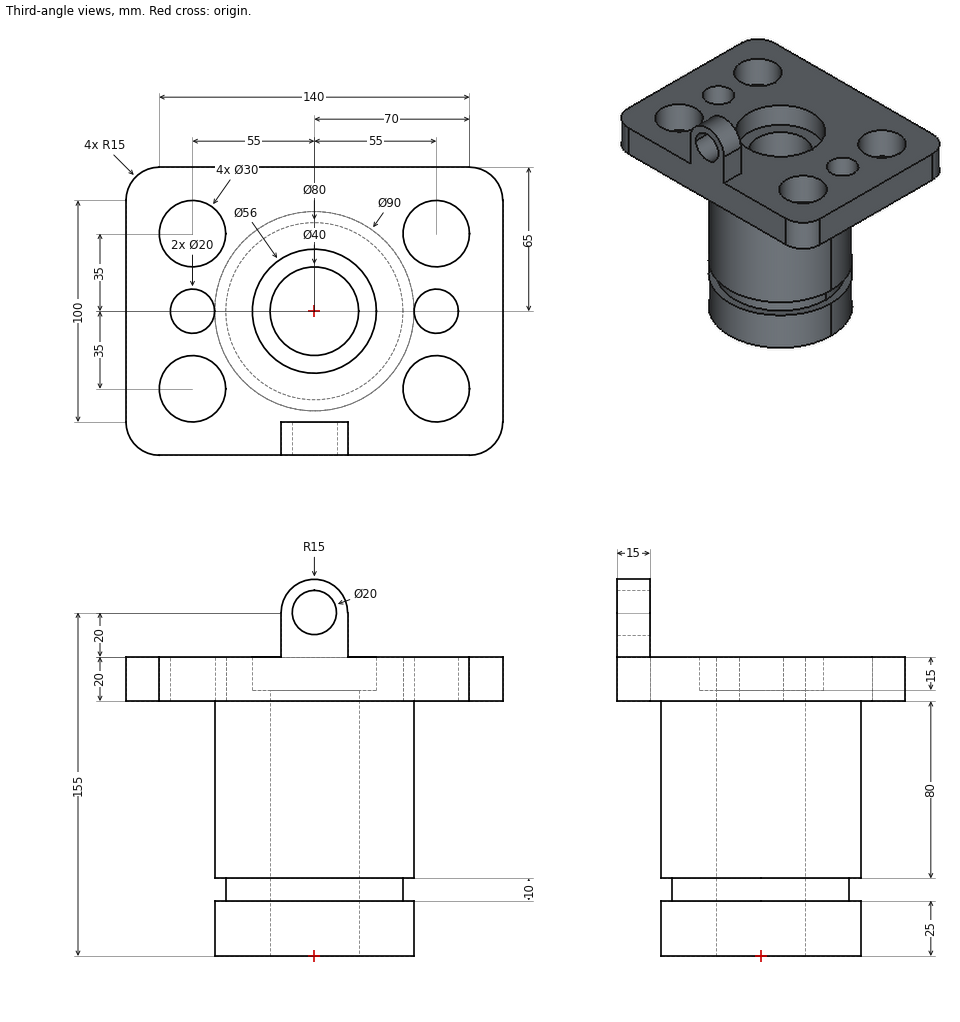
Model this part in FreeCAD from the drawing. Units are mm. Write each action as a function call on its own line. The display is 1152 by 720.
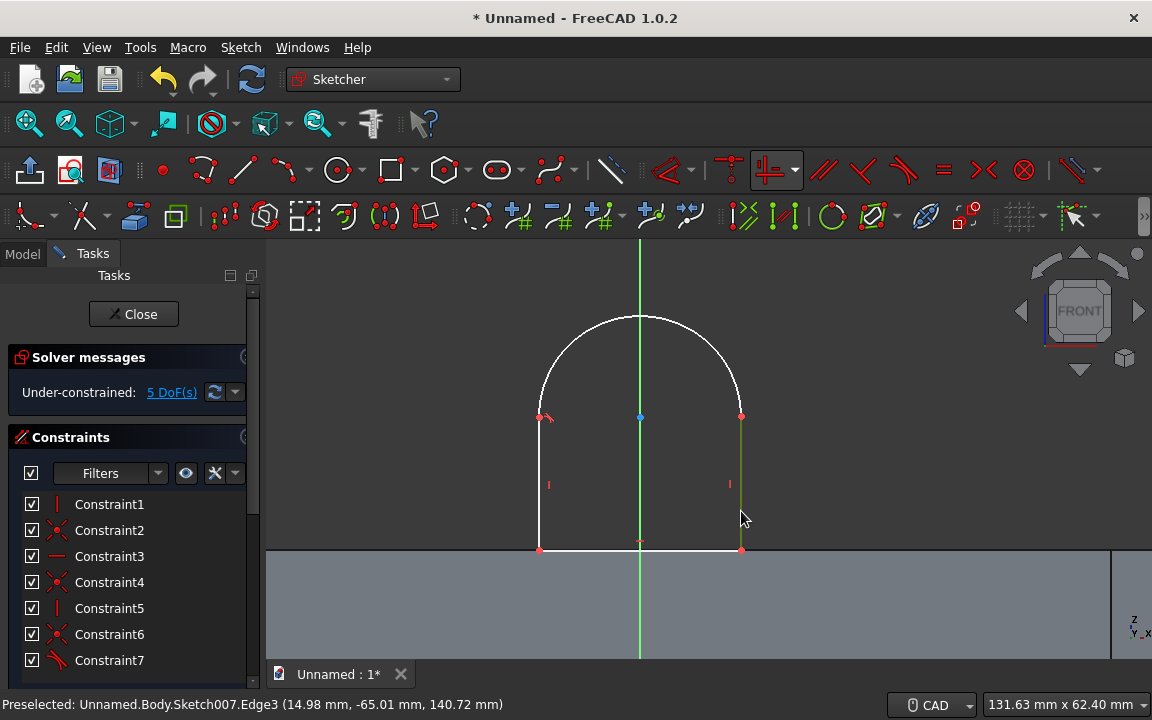
click(699, 335)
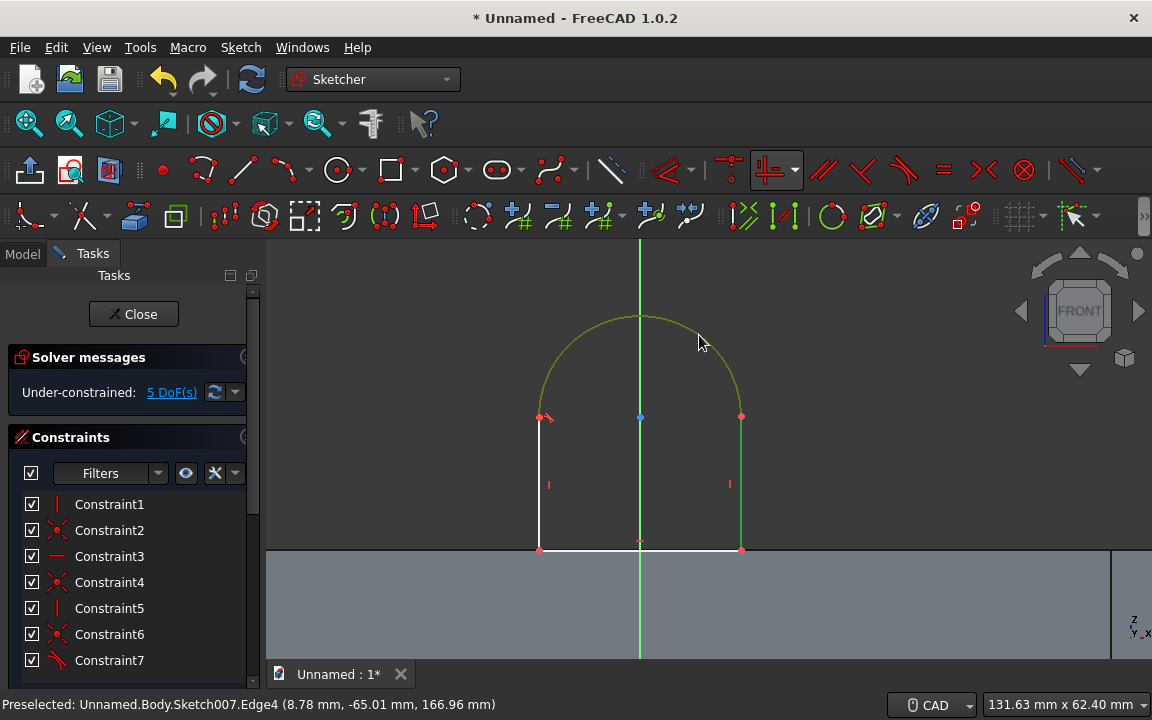
click(904, 170)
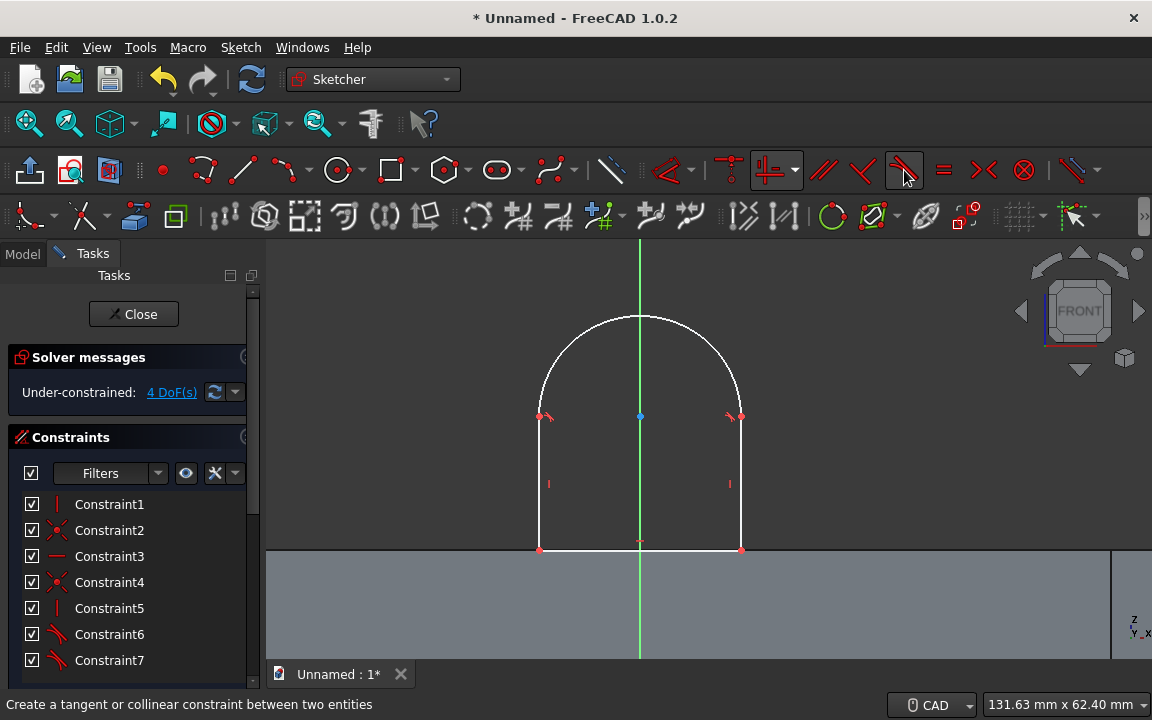
click(640, 417)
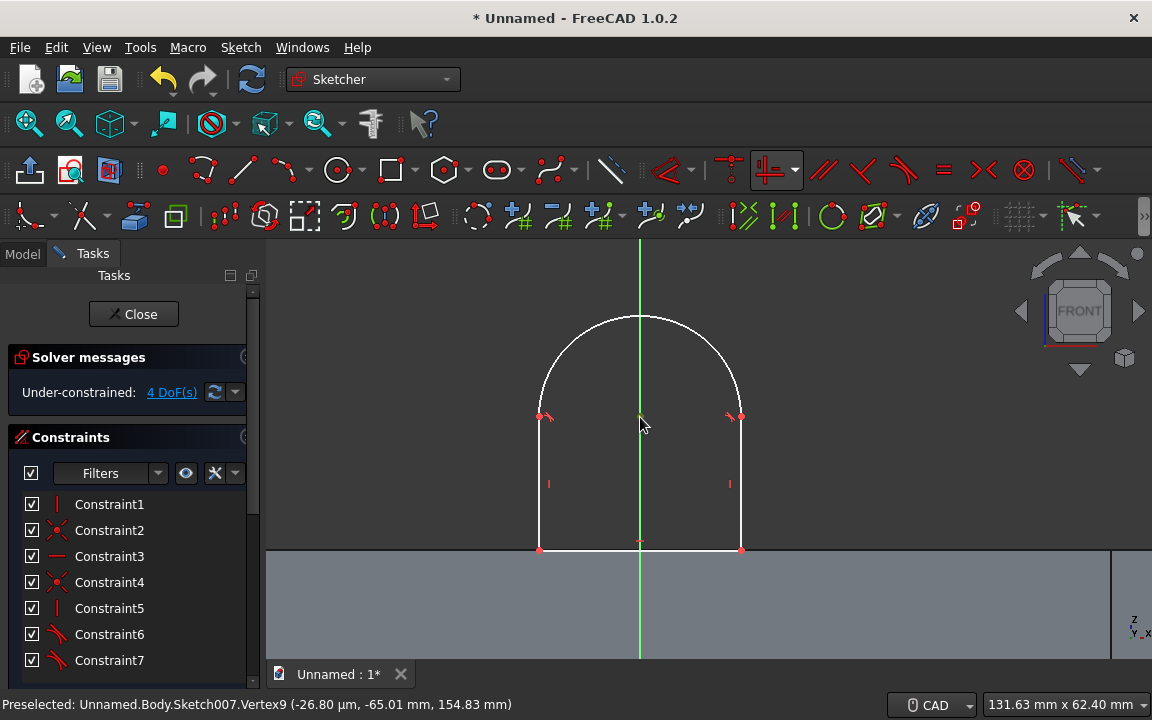
click(640, 605)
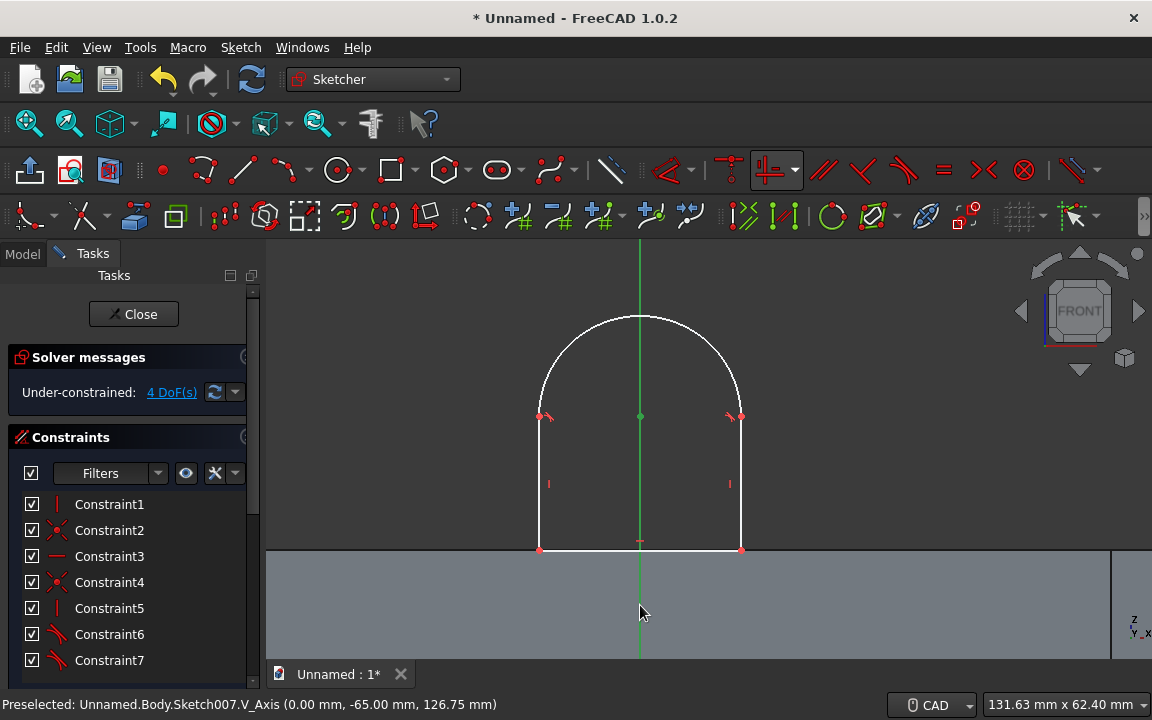
click(730, 170)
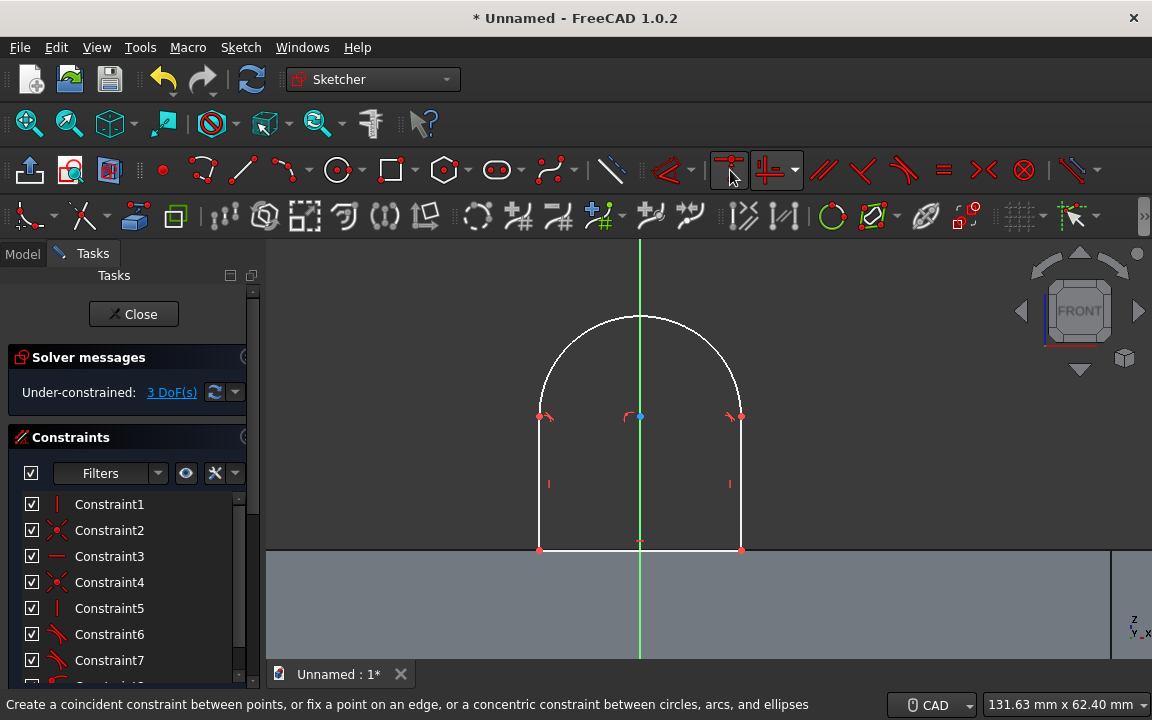
click(666, 170)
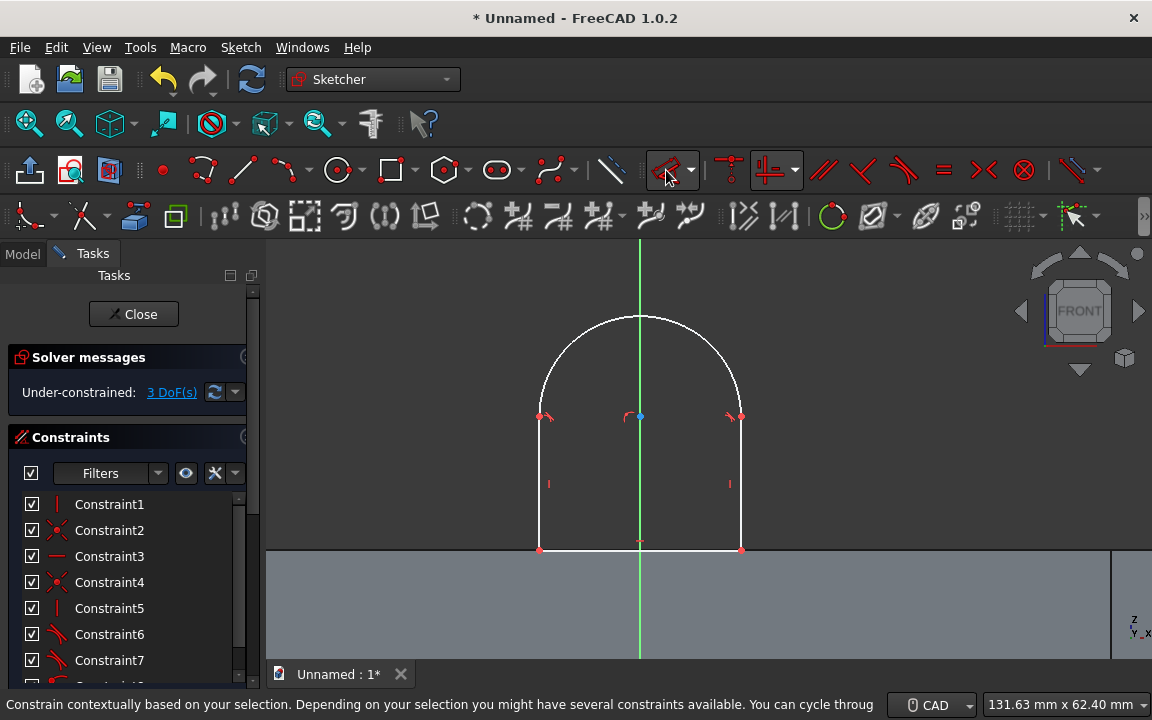
click(699, 335)
click(718, 309)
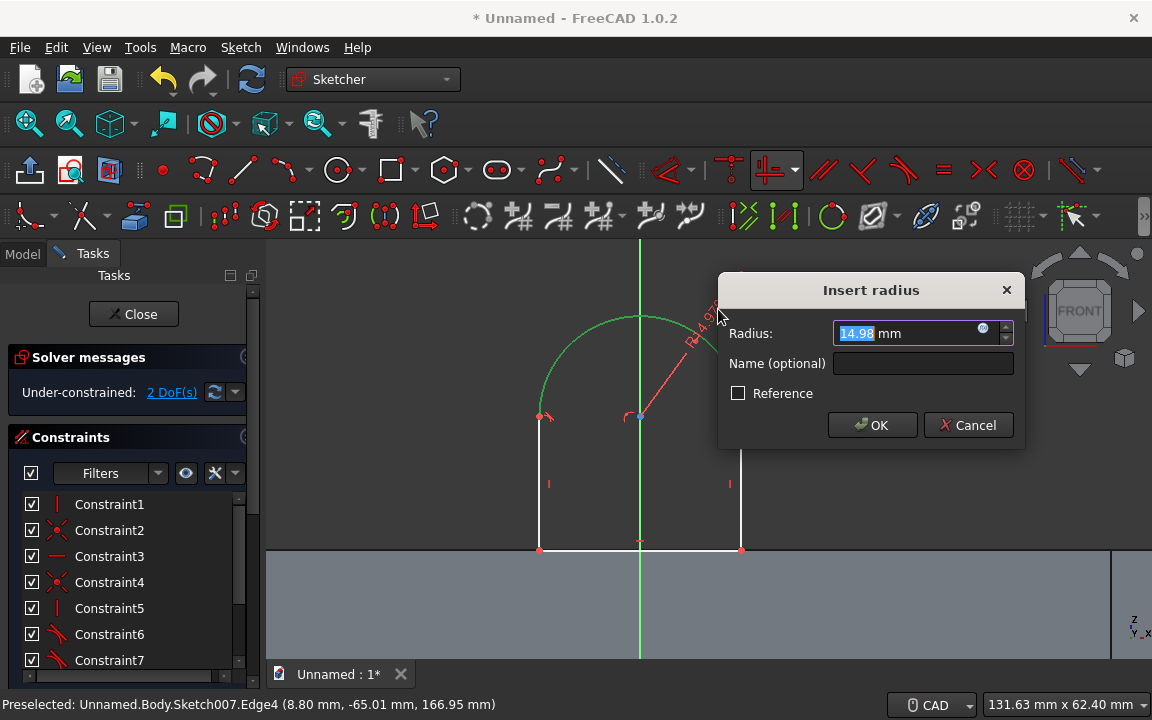
text(15)
key(Return)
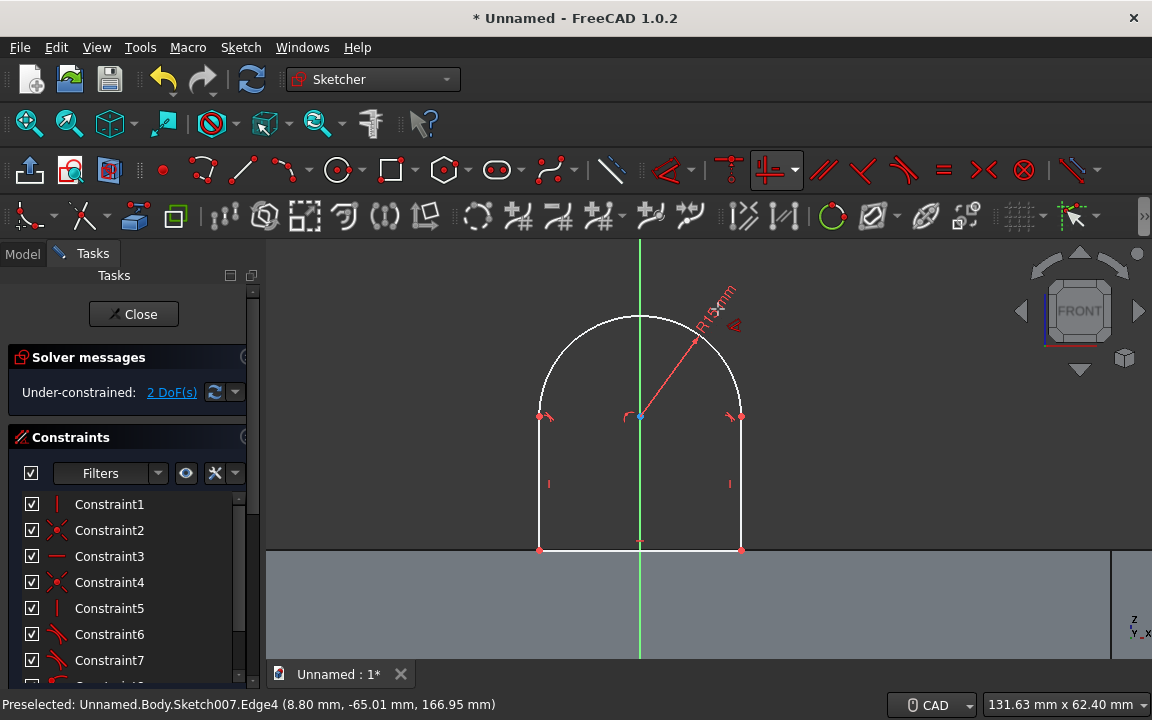
click(539, 457)
click(505, 484)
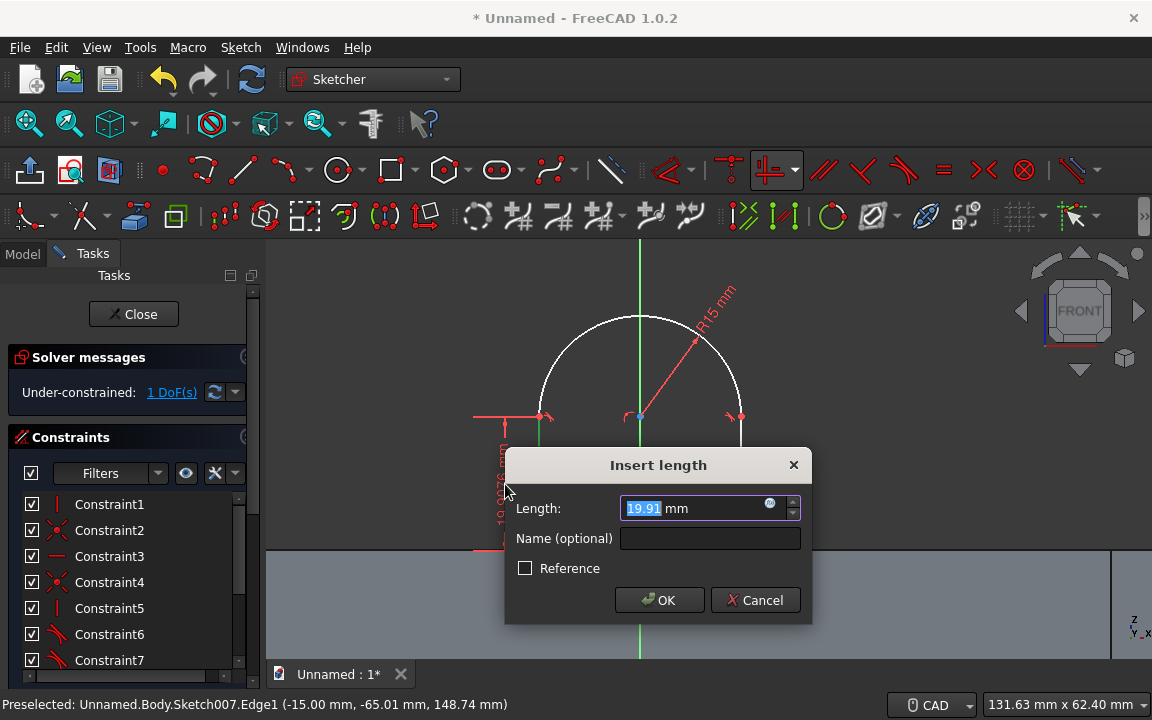
text(20)
key(Return)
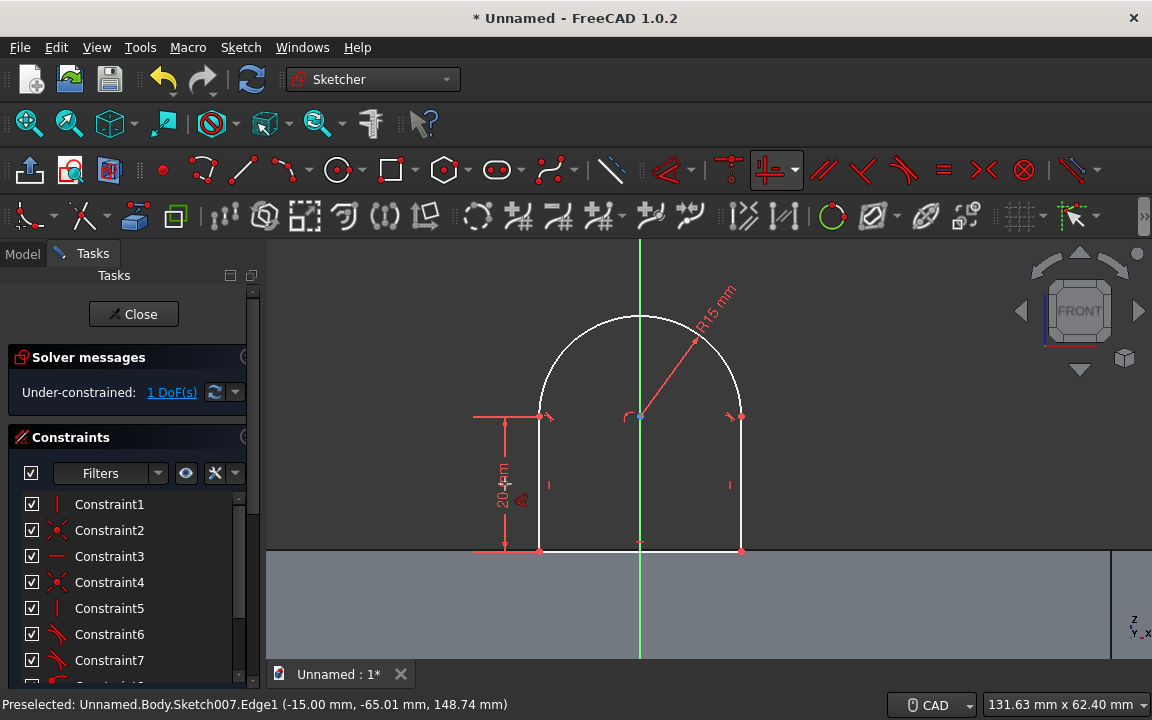
click(539, 417)
click(505, 524)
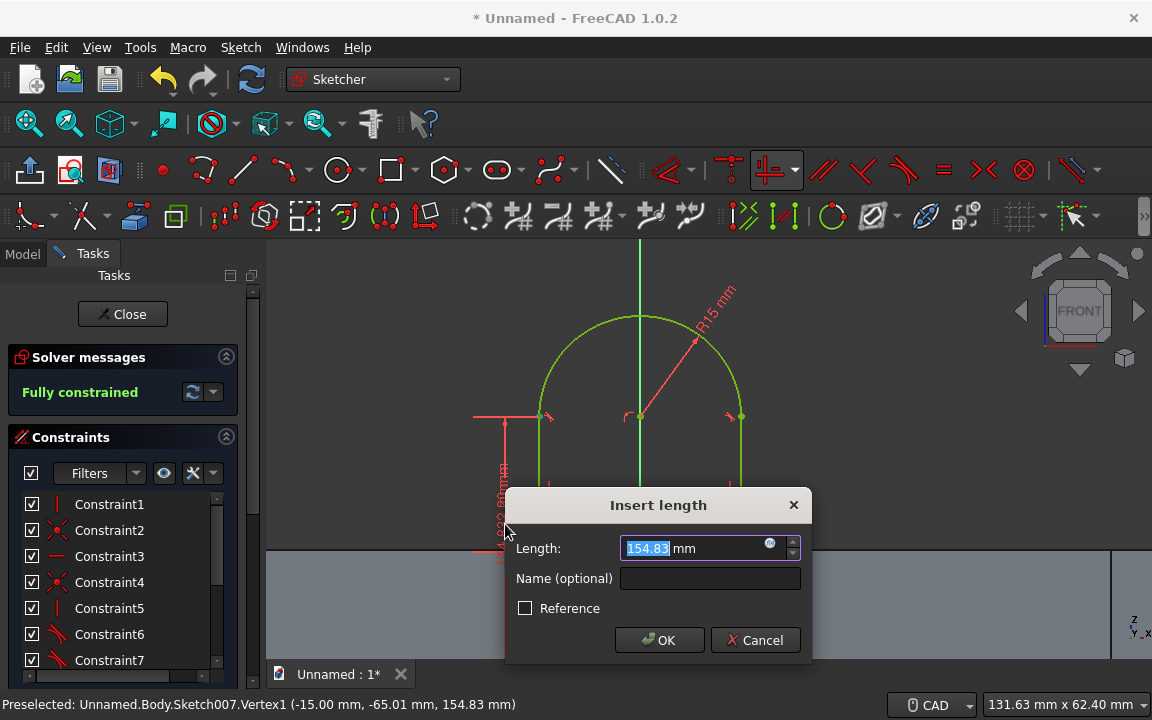
text(155)
key(Return)
key(Escape)